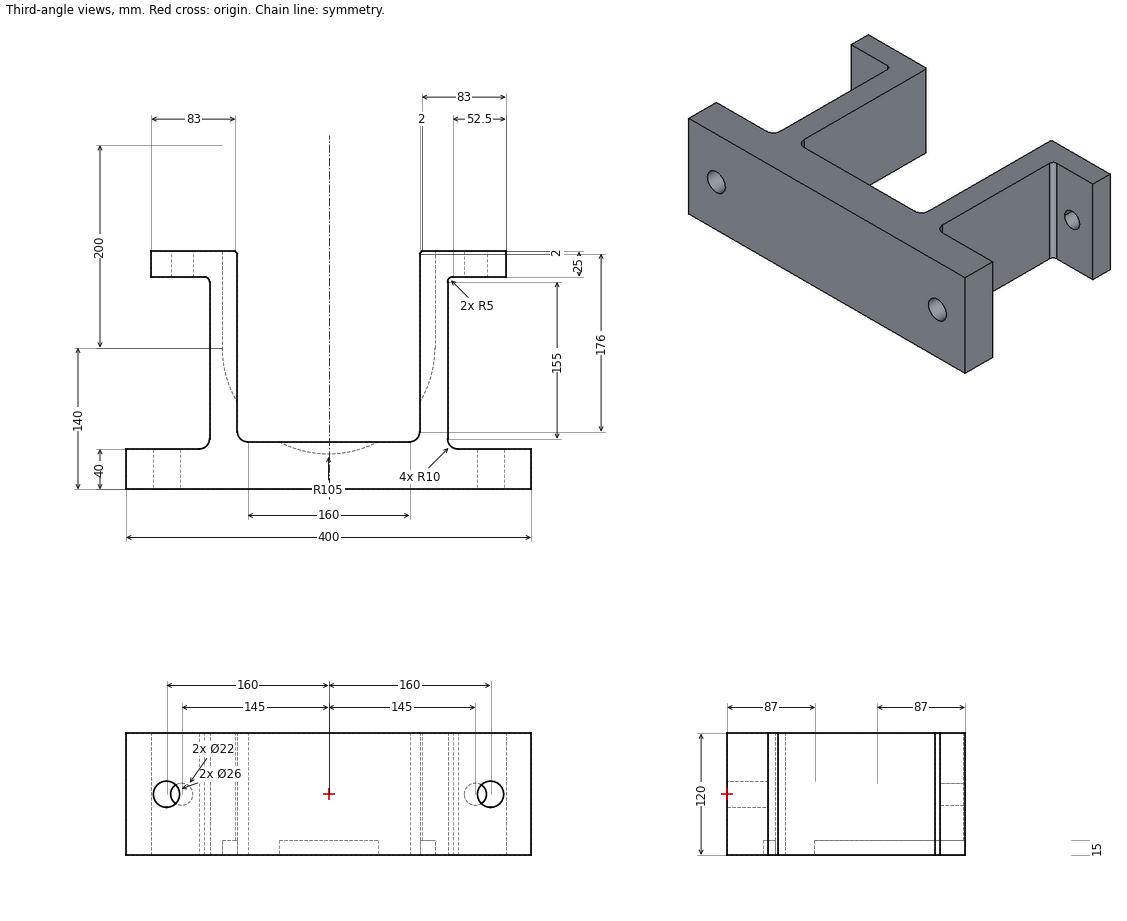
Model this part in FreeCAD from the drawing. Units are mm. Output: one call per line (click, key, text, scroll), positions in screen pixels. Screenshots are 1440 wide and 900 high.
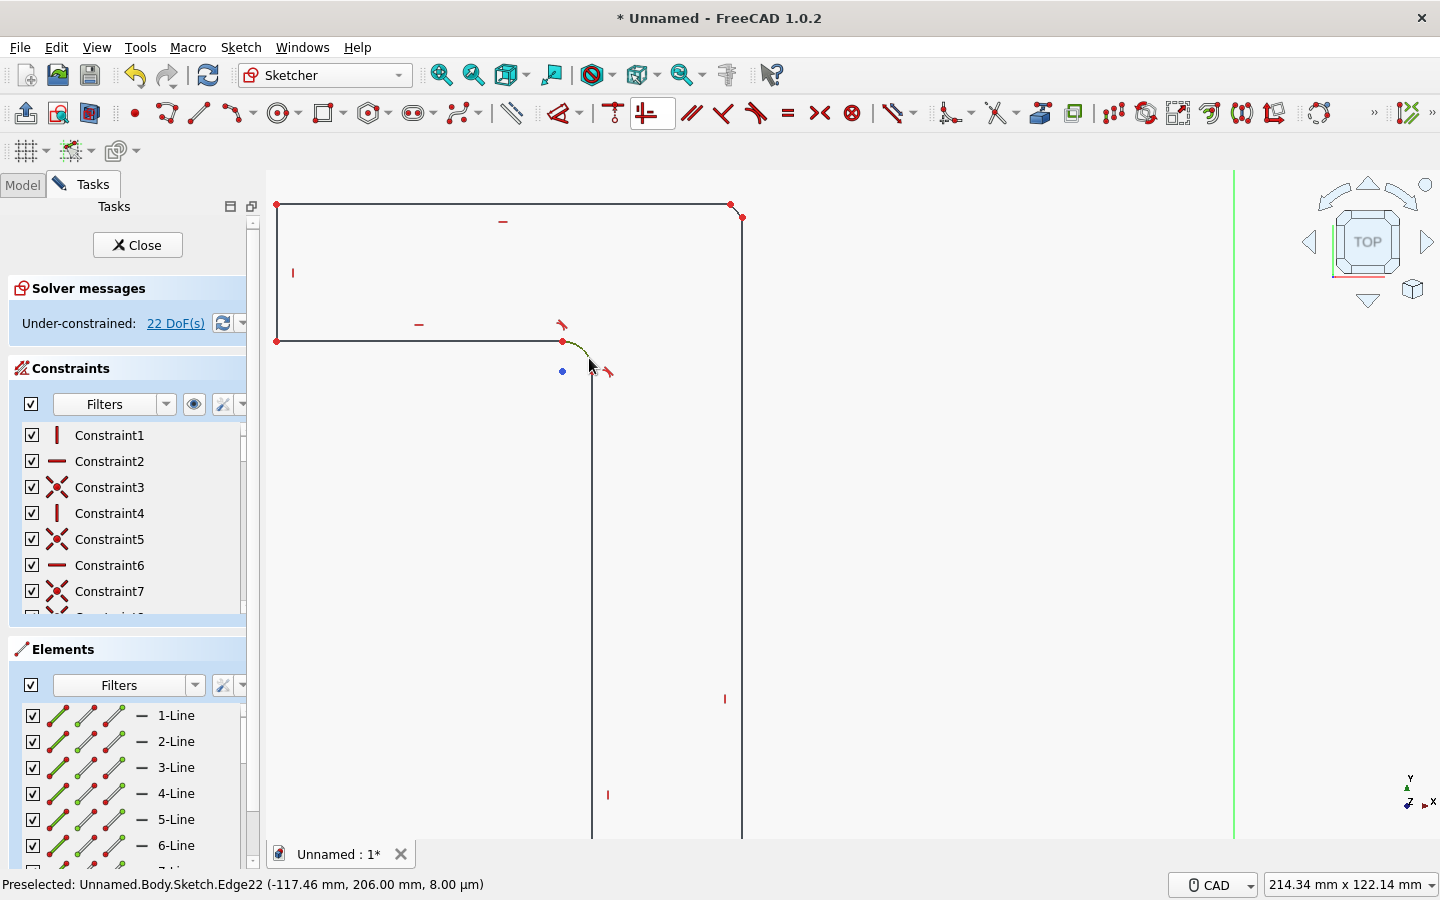
key(e)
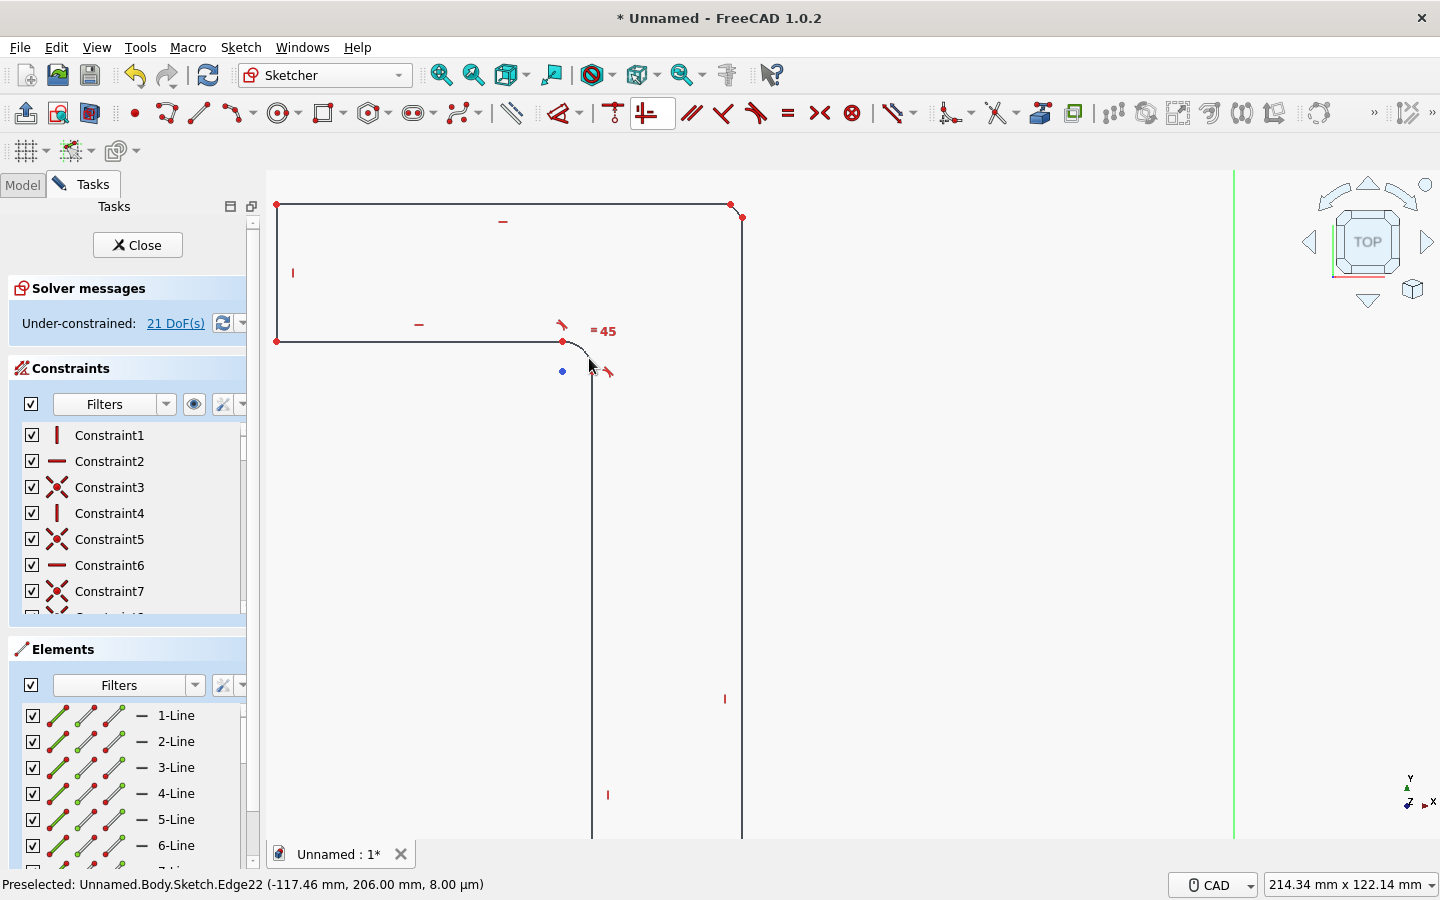
scroll(591, 357, down, 6)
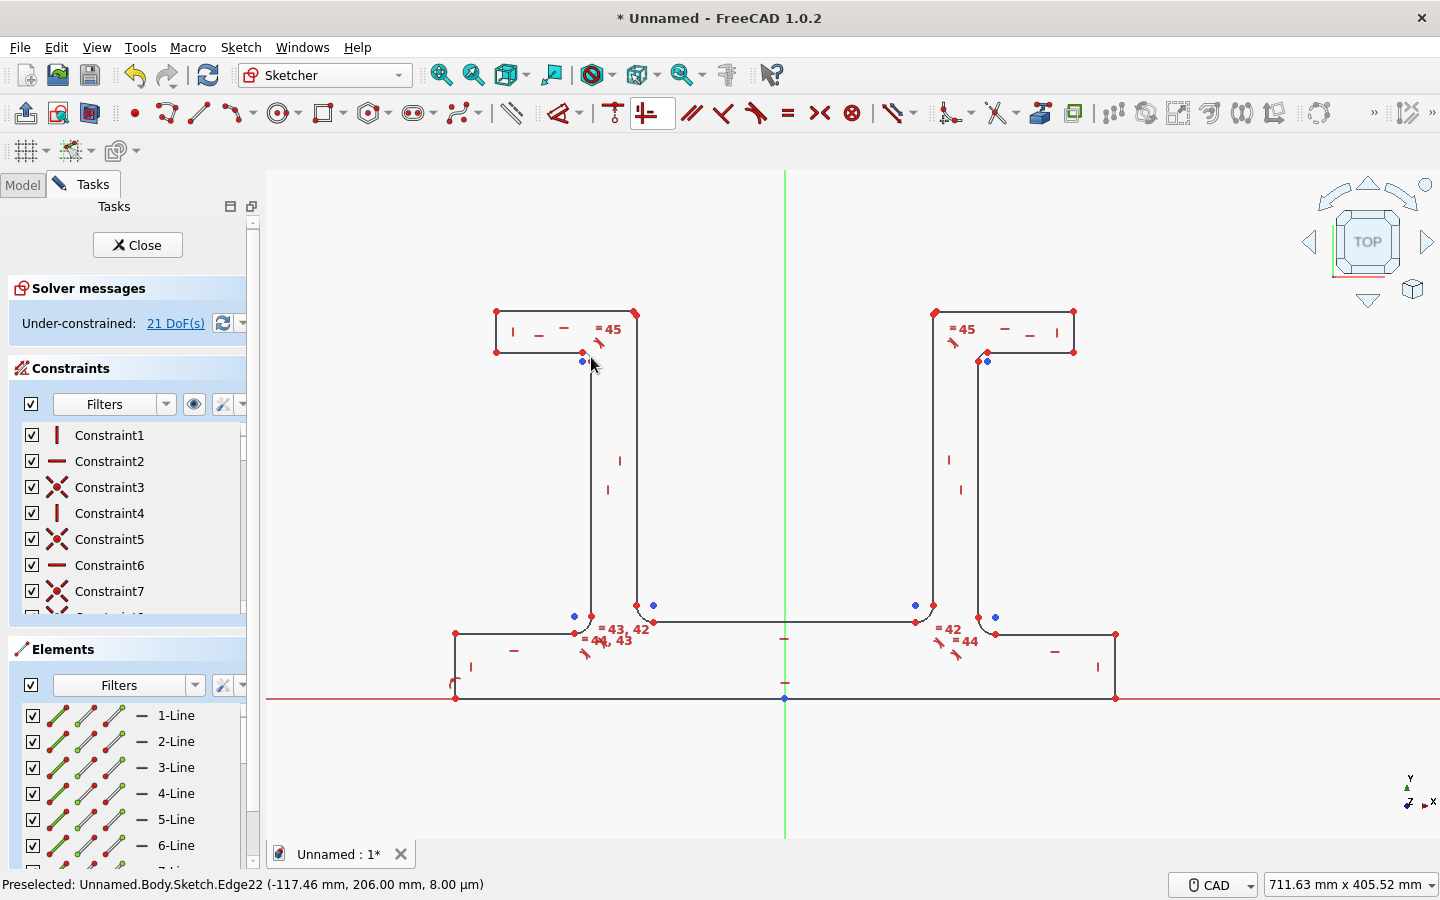
scroll(987, 362, up, 2)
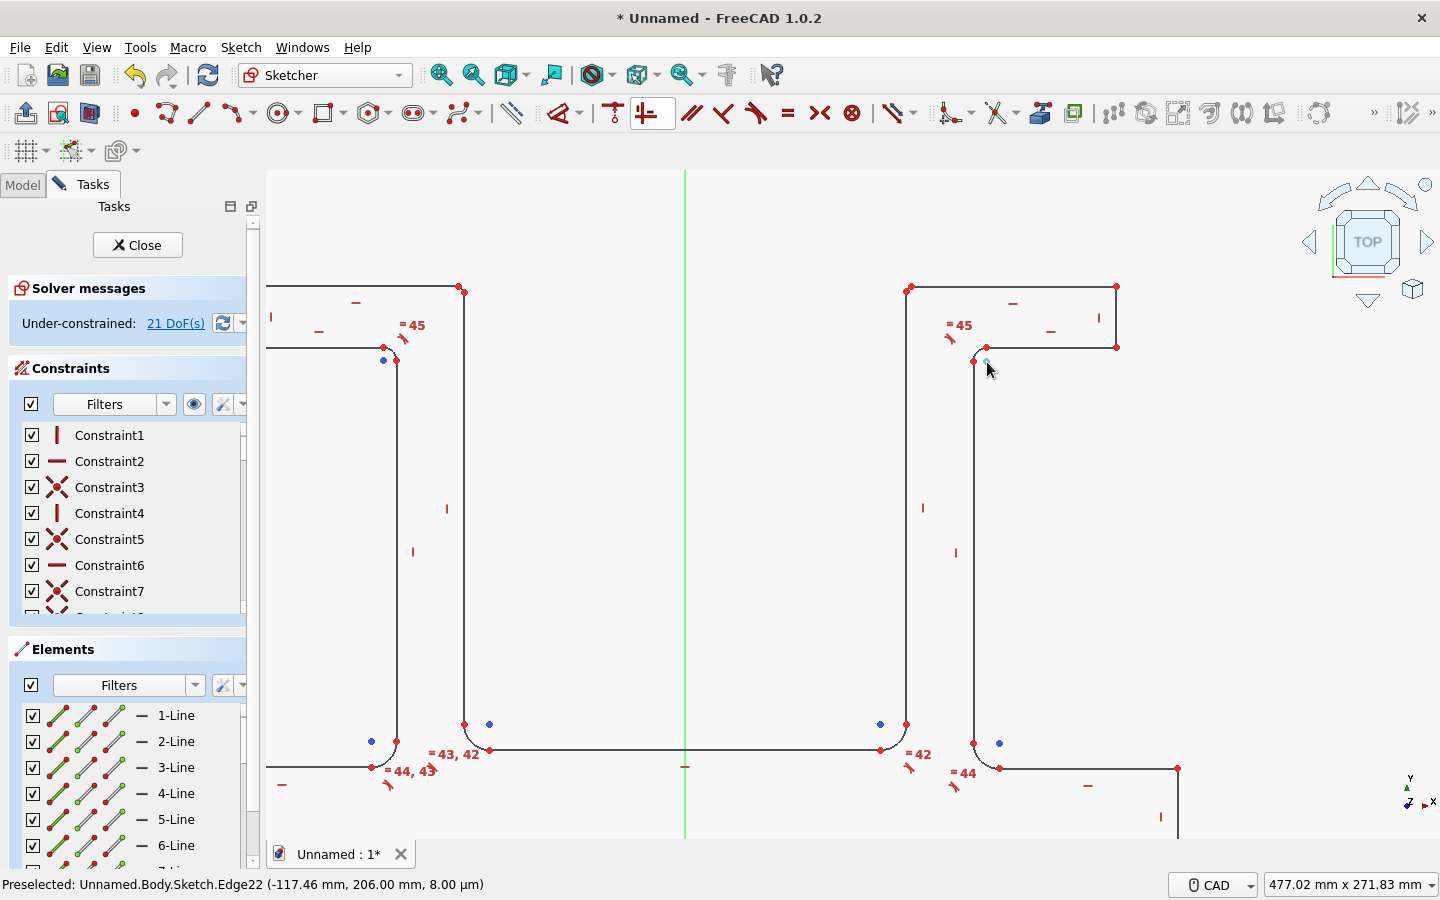
click(987, 361)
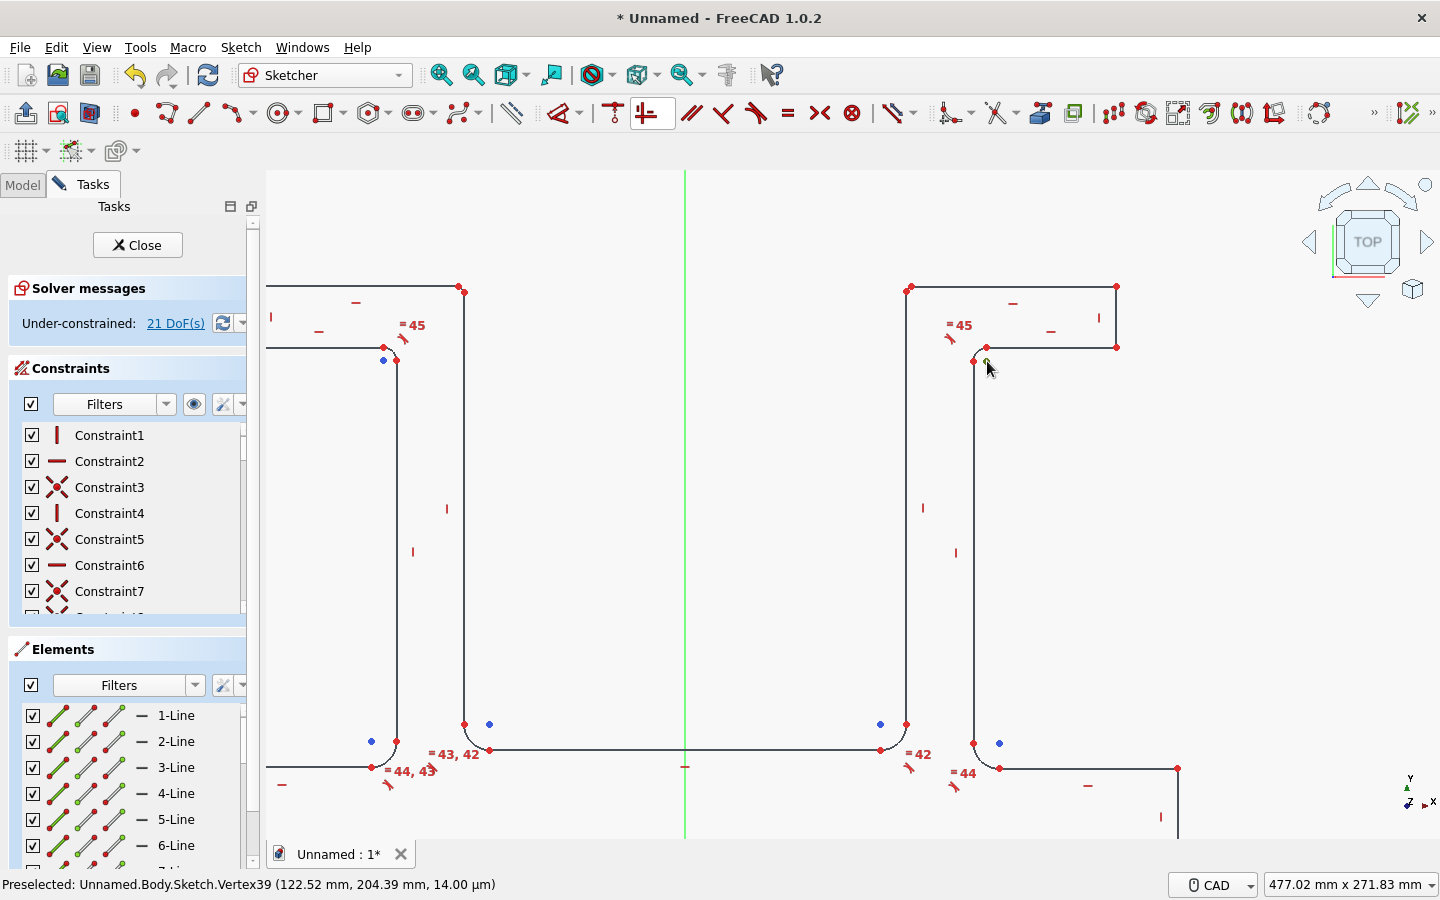
click(383, 361)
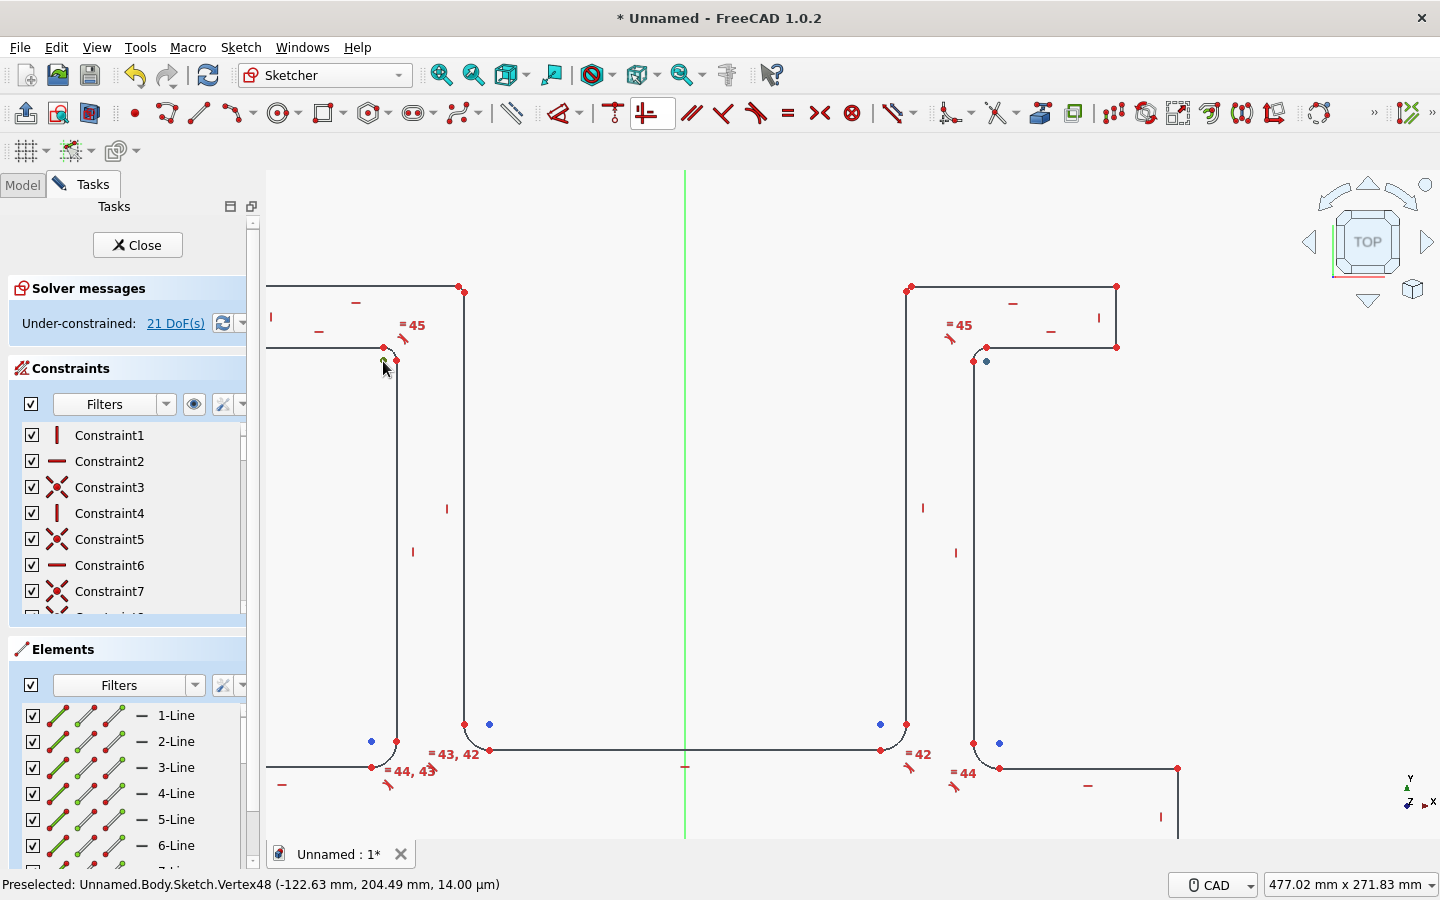
click(685, 680)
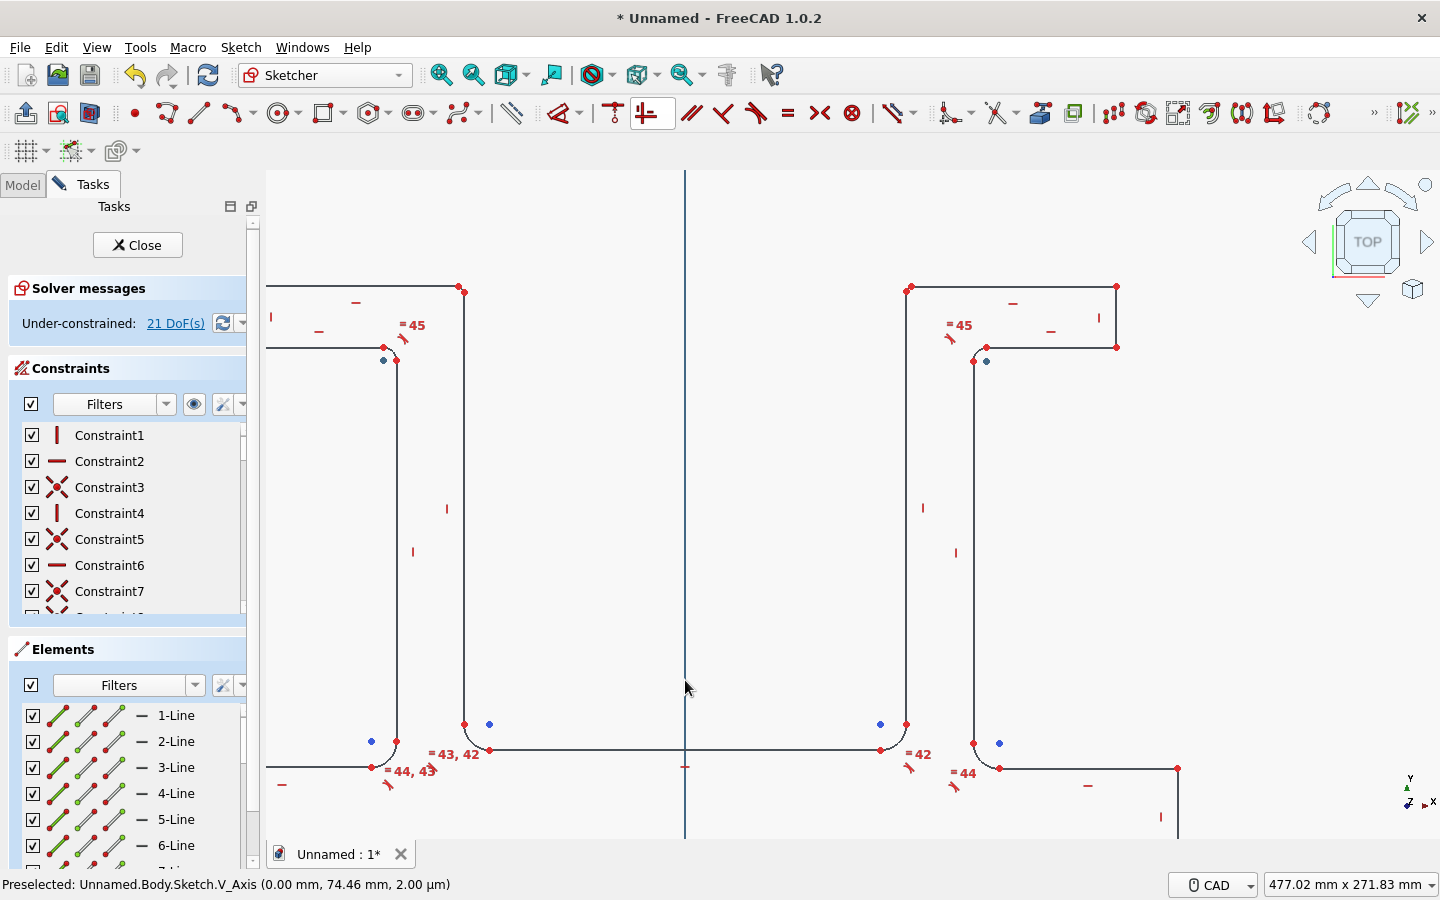
key(s)